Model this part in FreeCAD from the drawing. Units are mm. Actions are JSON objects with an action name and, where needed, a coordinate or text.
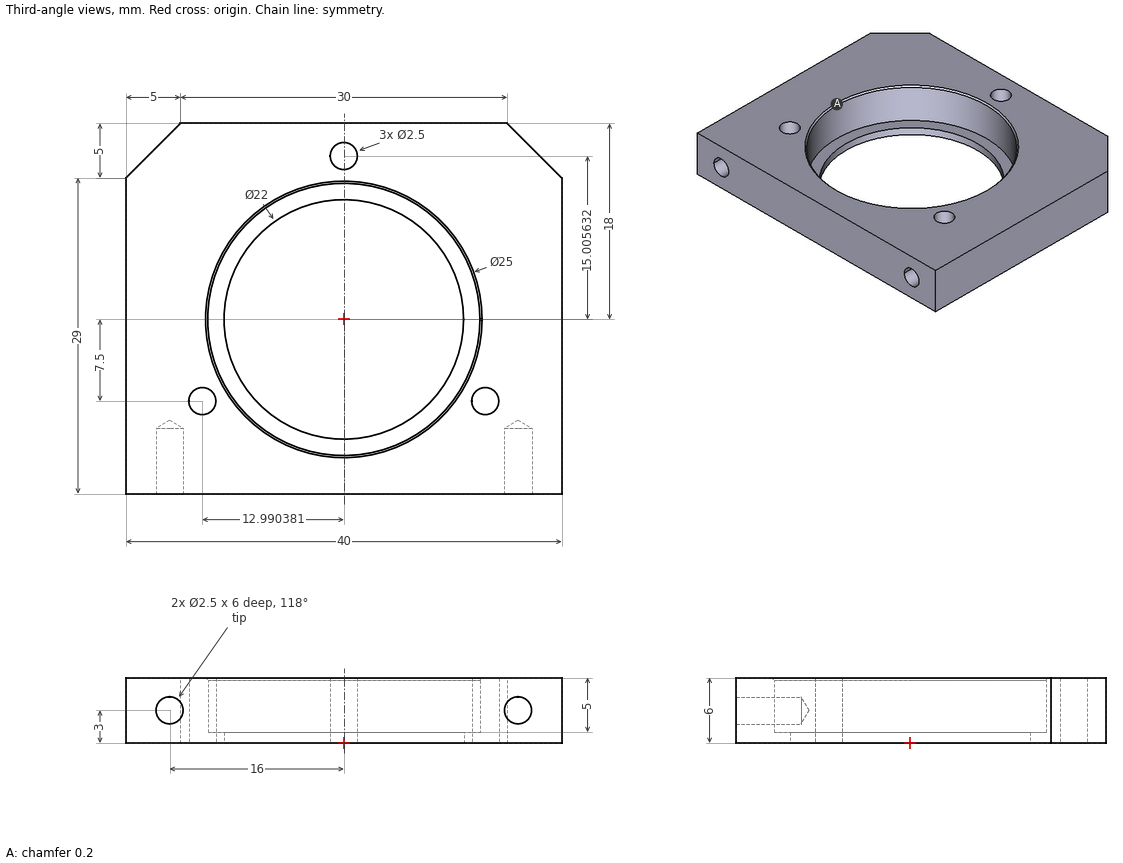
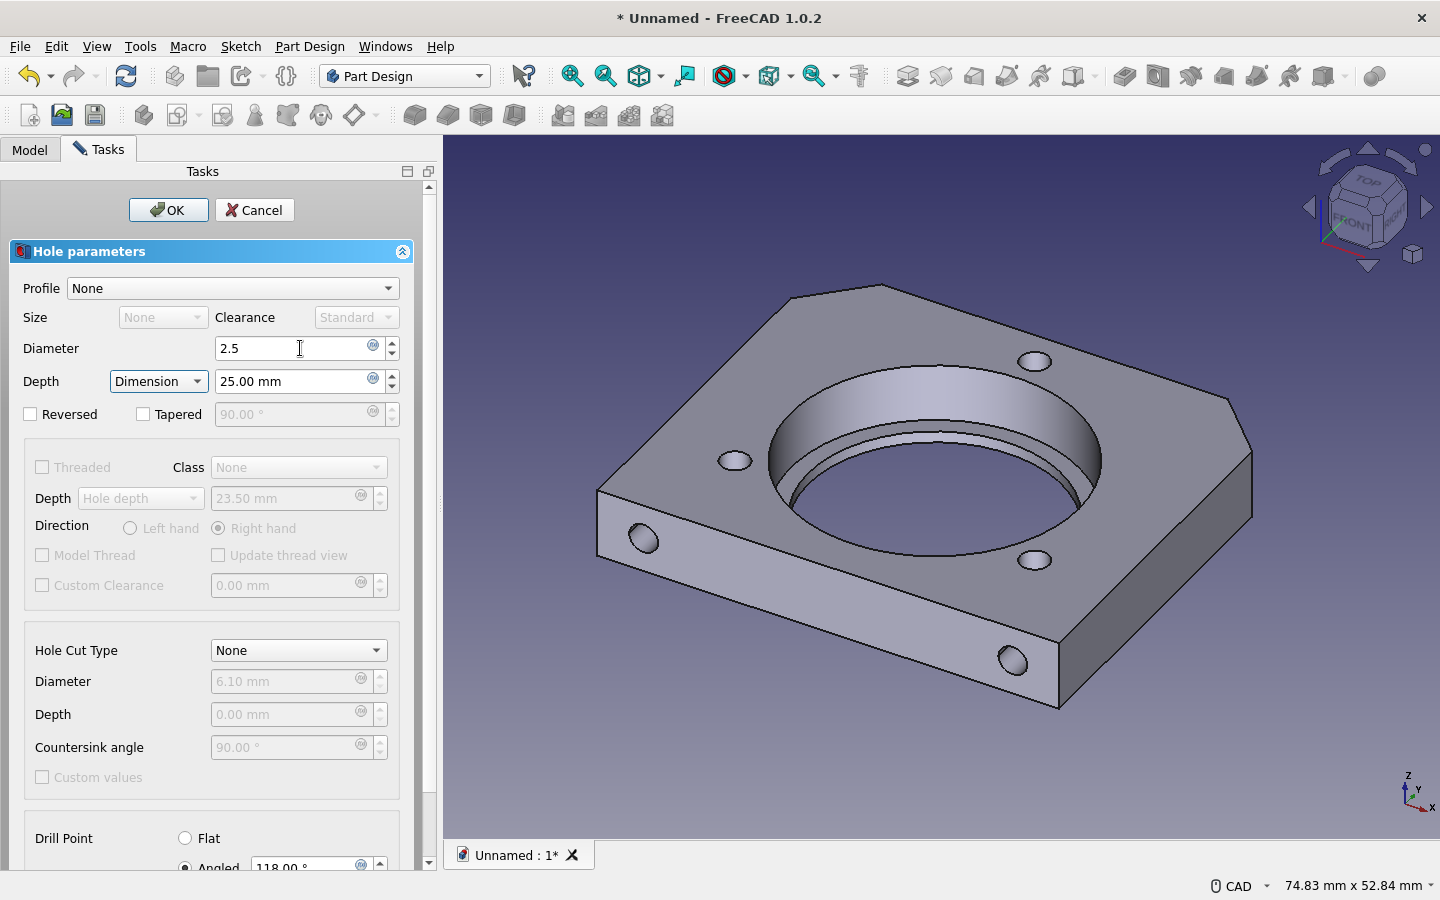
{"action": "triple_click", "coordinate": [300, 382]}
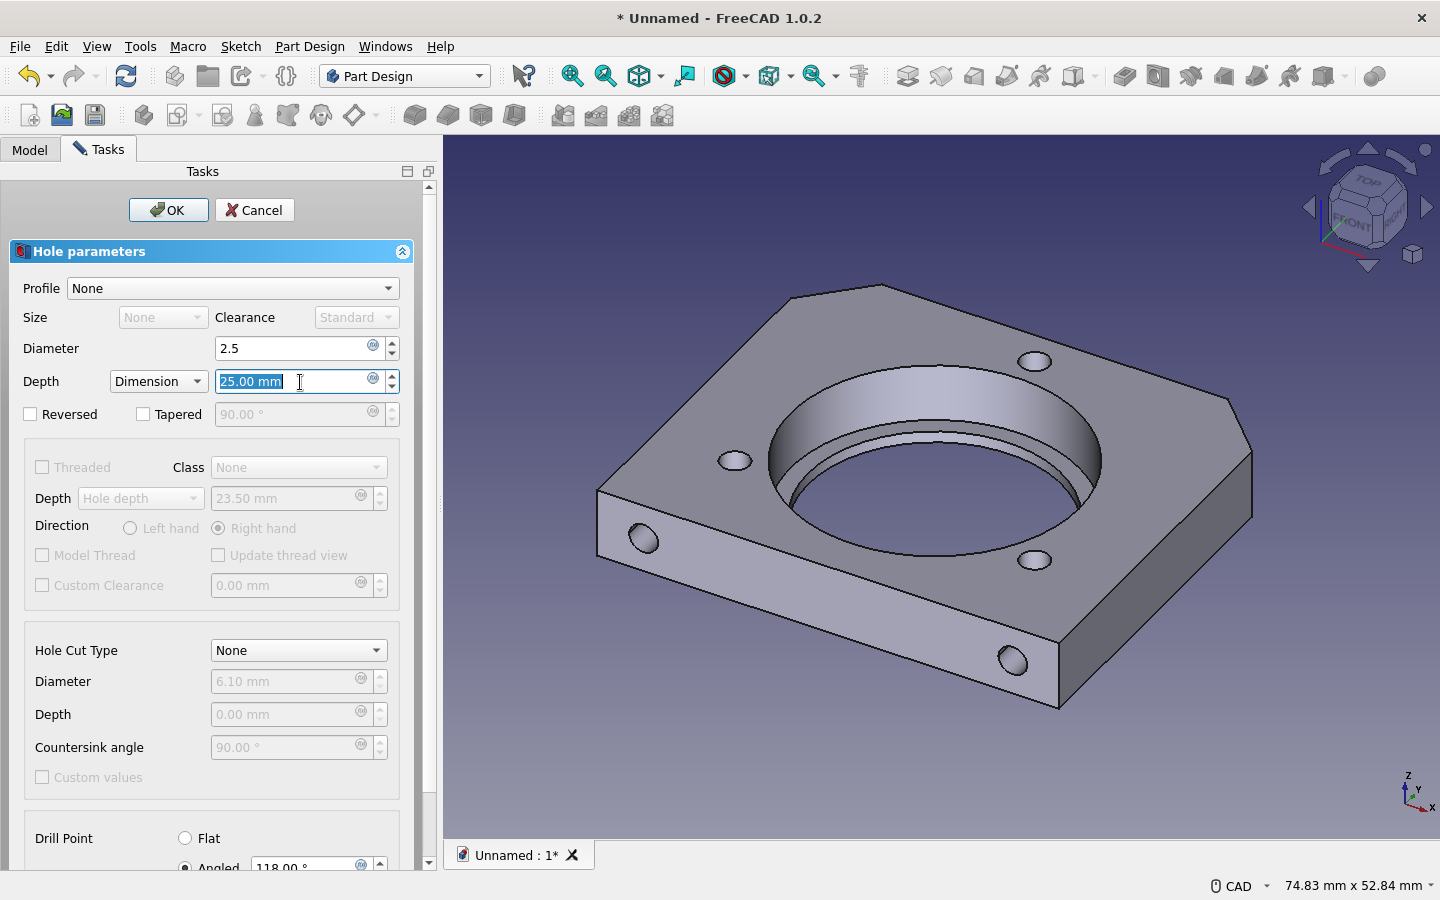
{"action": "type", "text": "6"}
{"action": "key", "text": "Tab"}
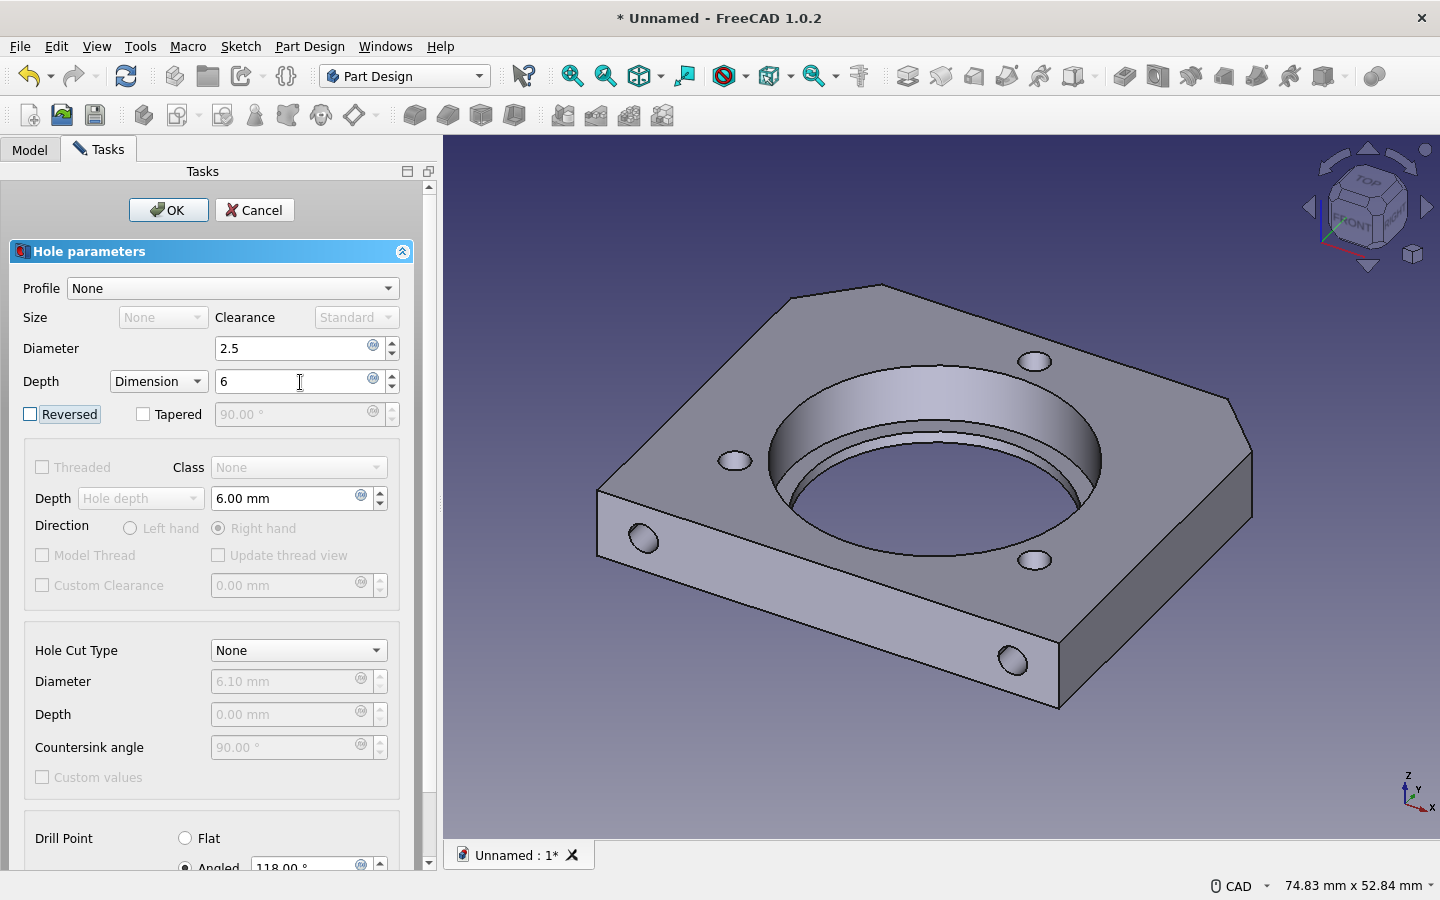
{"action": "left_click", "coordinate": [169, 210]}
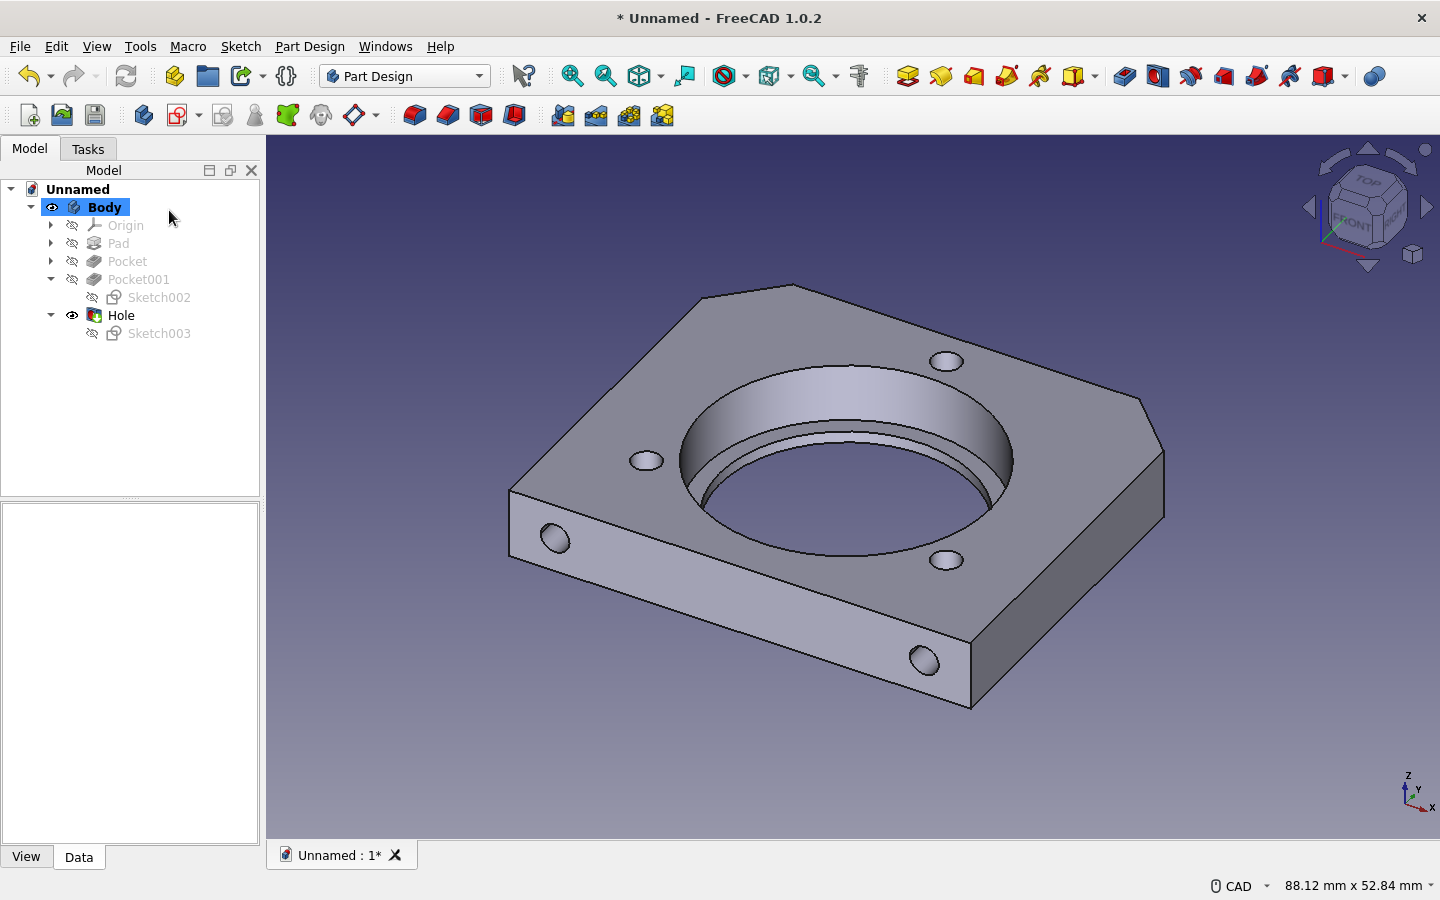
{"action": "left_click", "coordinate": [702, 412]}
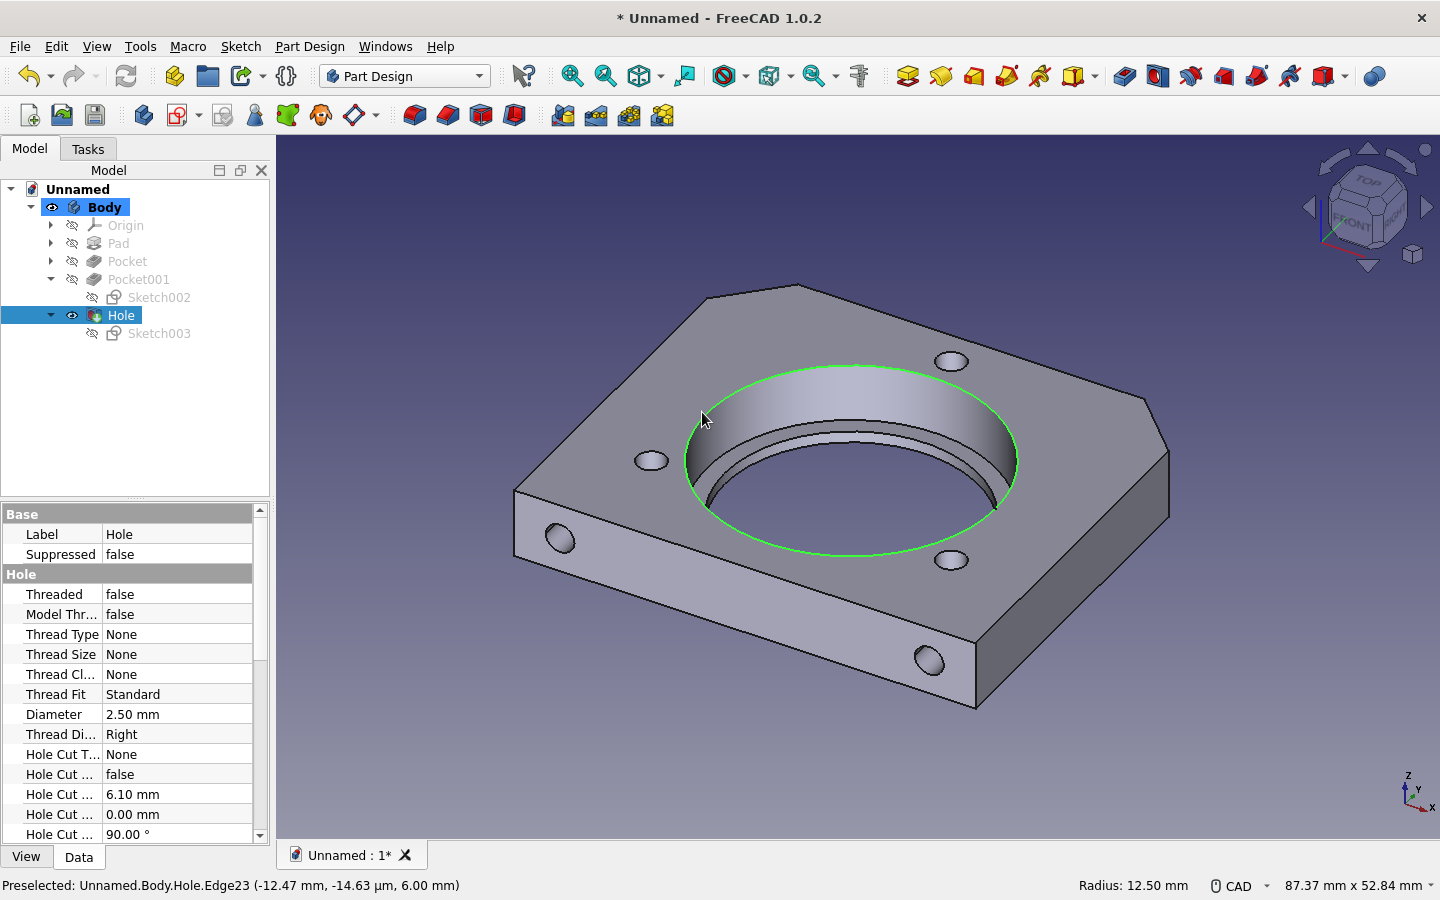
{"action": "left_click", "coordinate": [448, 116]}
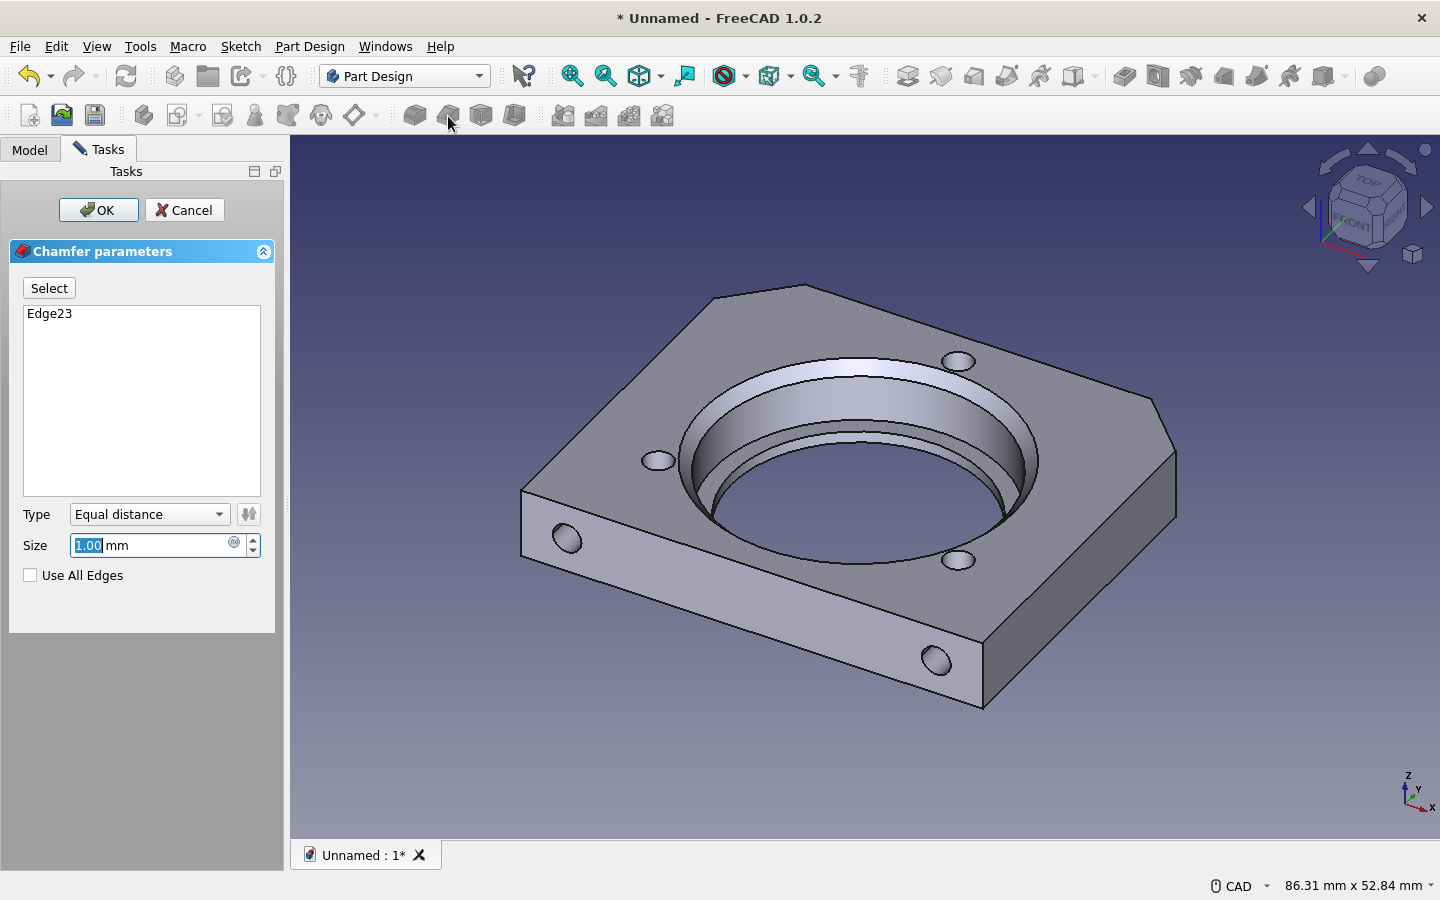
{"action": "type", "text": "0.2"}
{"action": "key", "text": "Tab"}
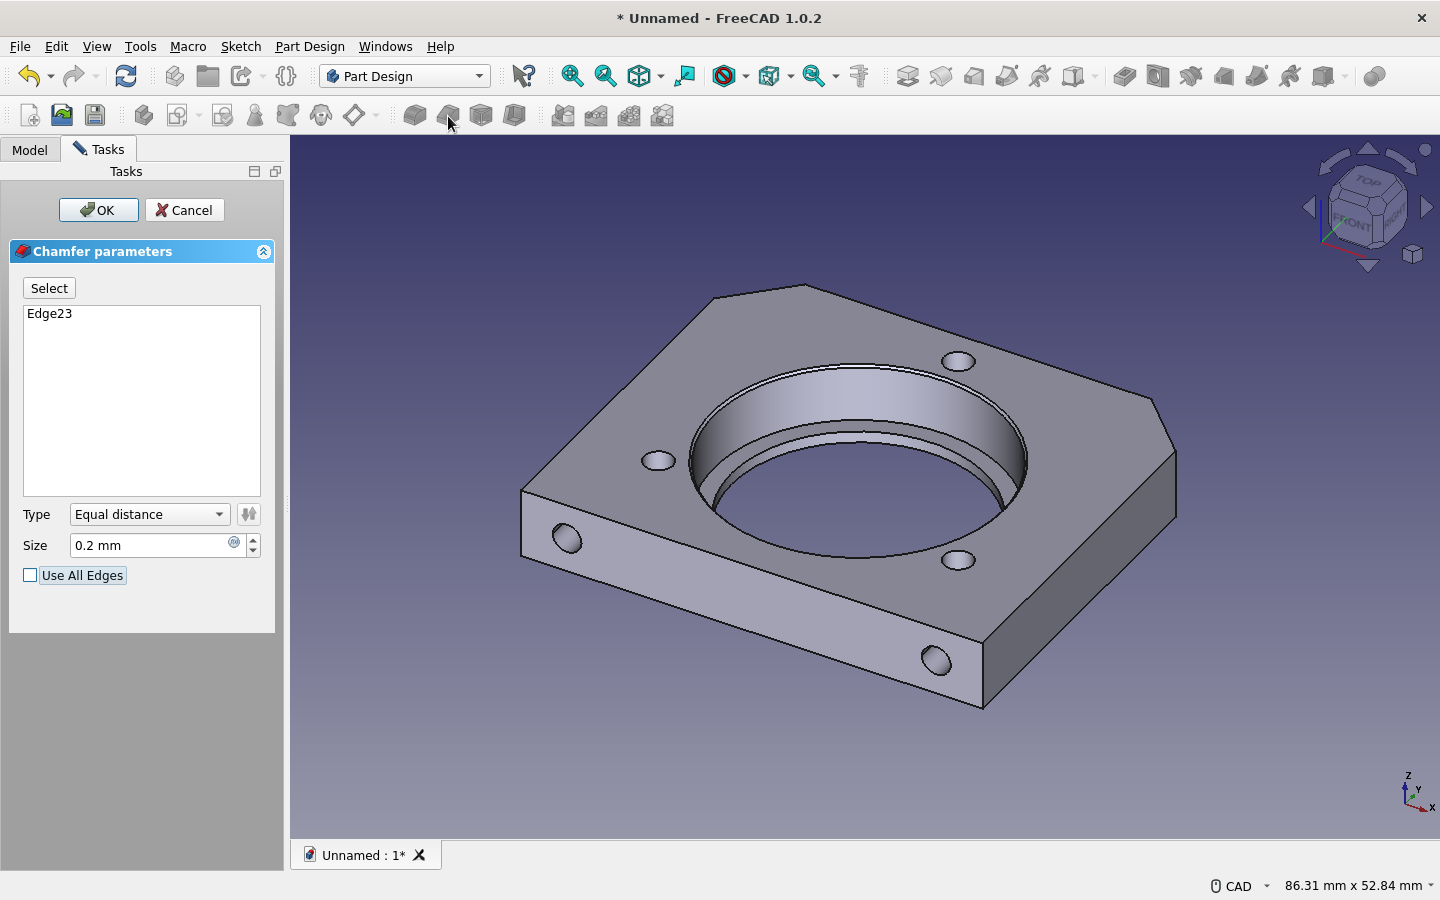
{"action": "left_click", "coordinate": [99, 210]}